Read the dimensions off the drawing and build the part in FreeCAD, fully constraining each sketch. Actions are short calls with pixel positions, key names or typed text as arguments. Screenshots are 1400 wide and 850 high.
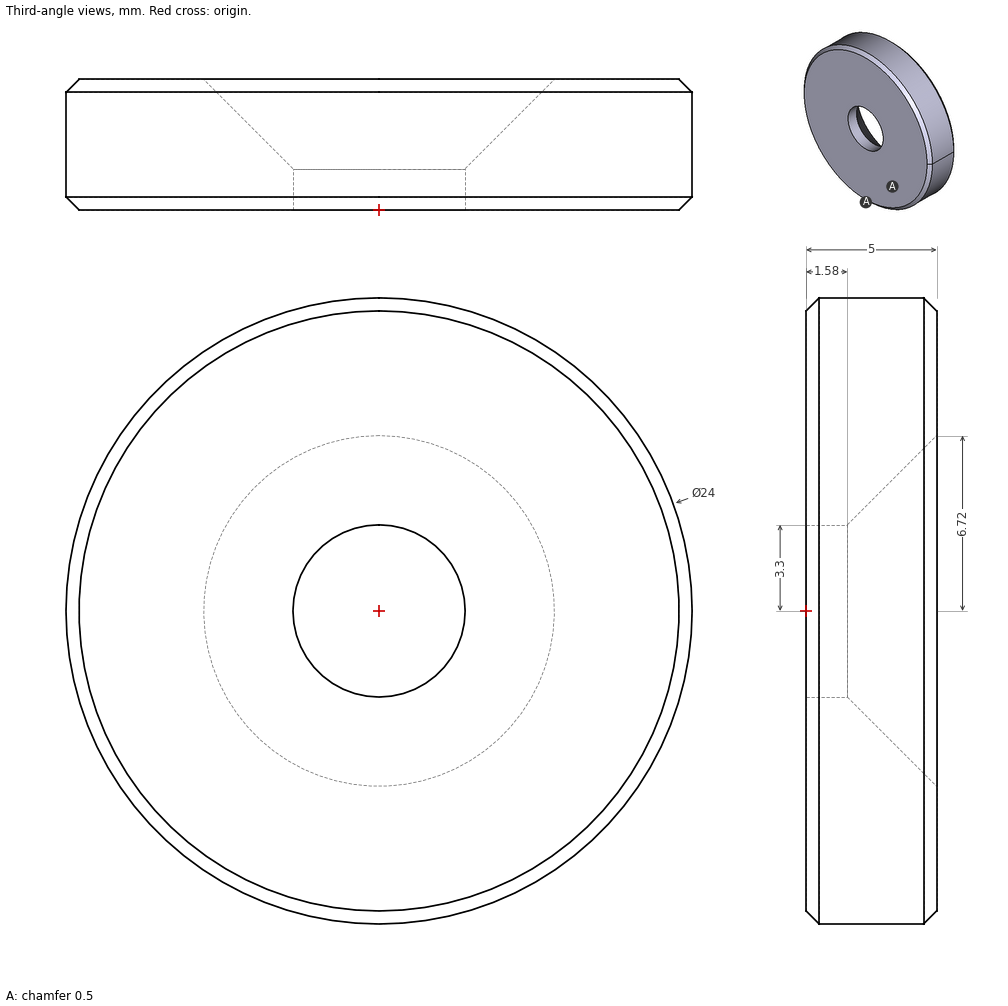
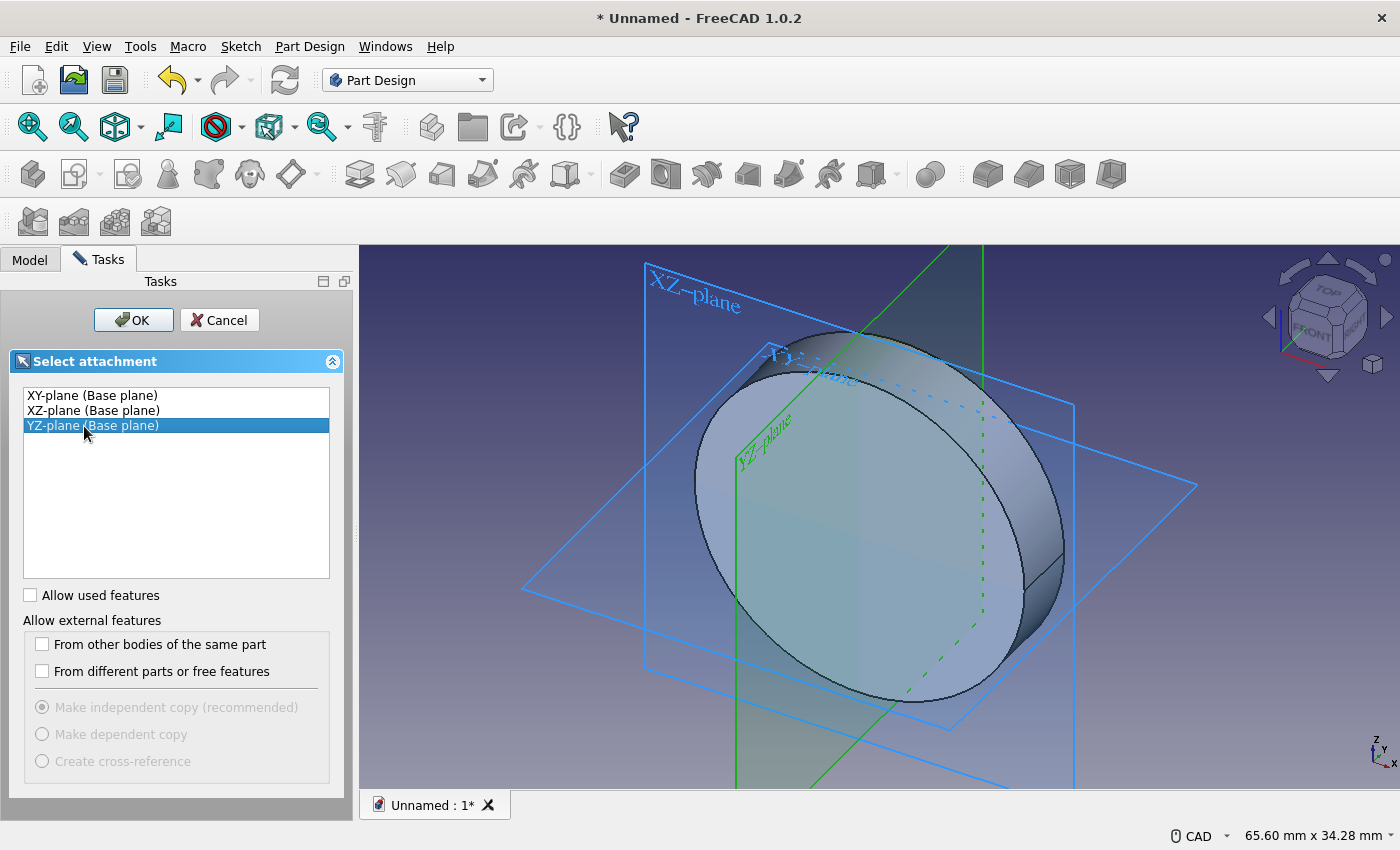
click(134, 320)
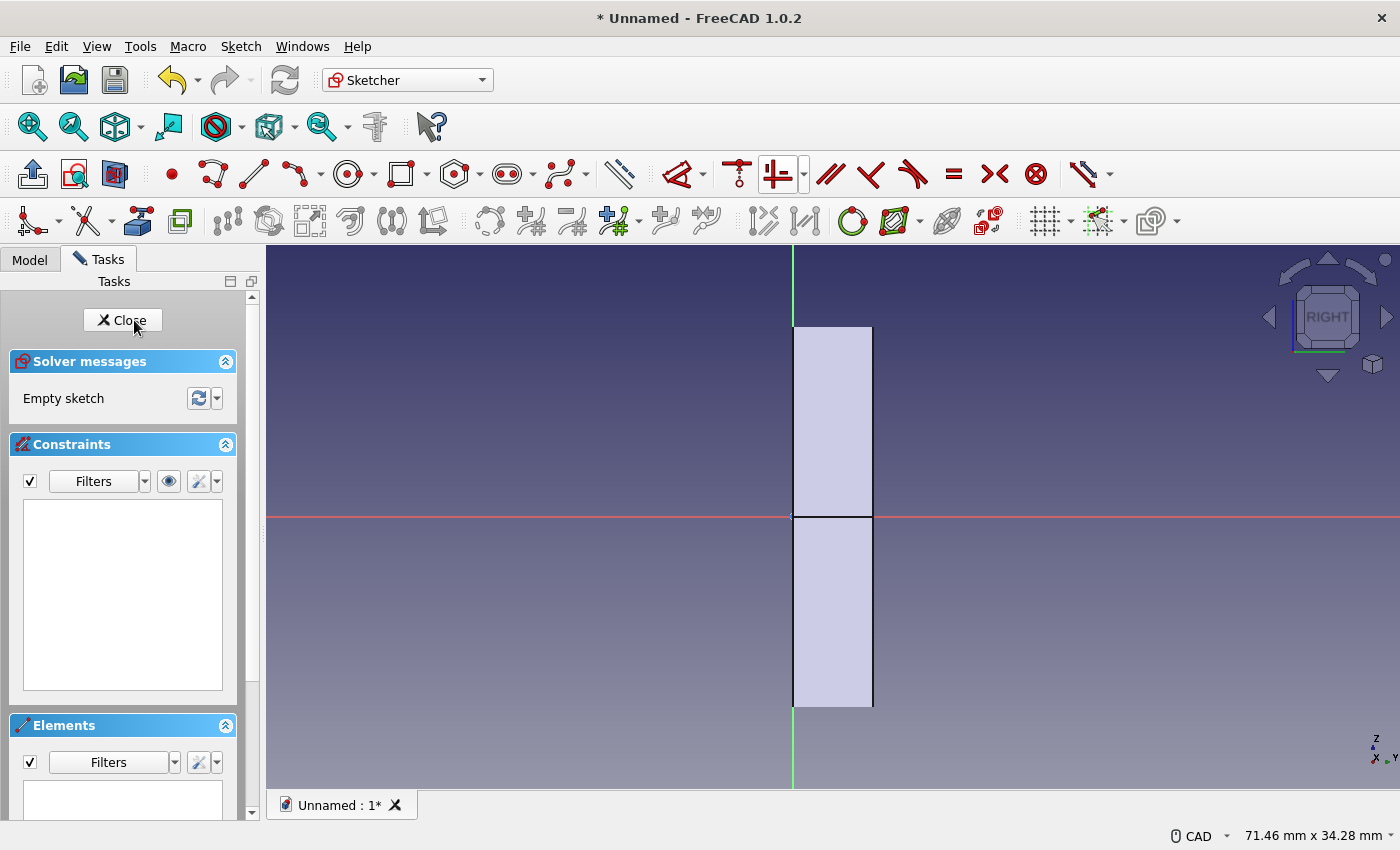
click(115, 174)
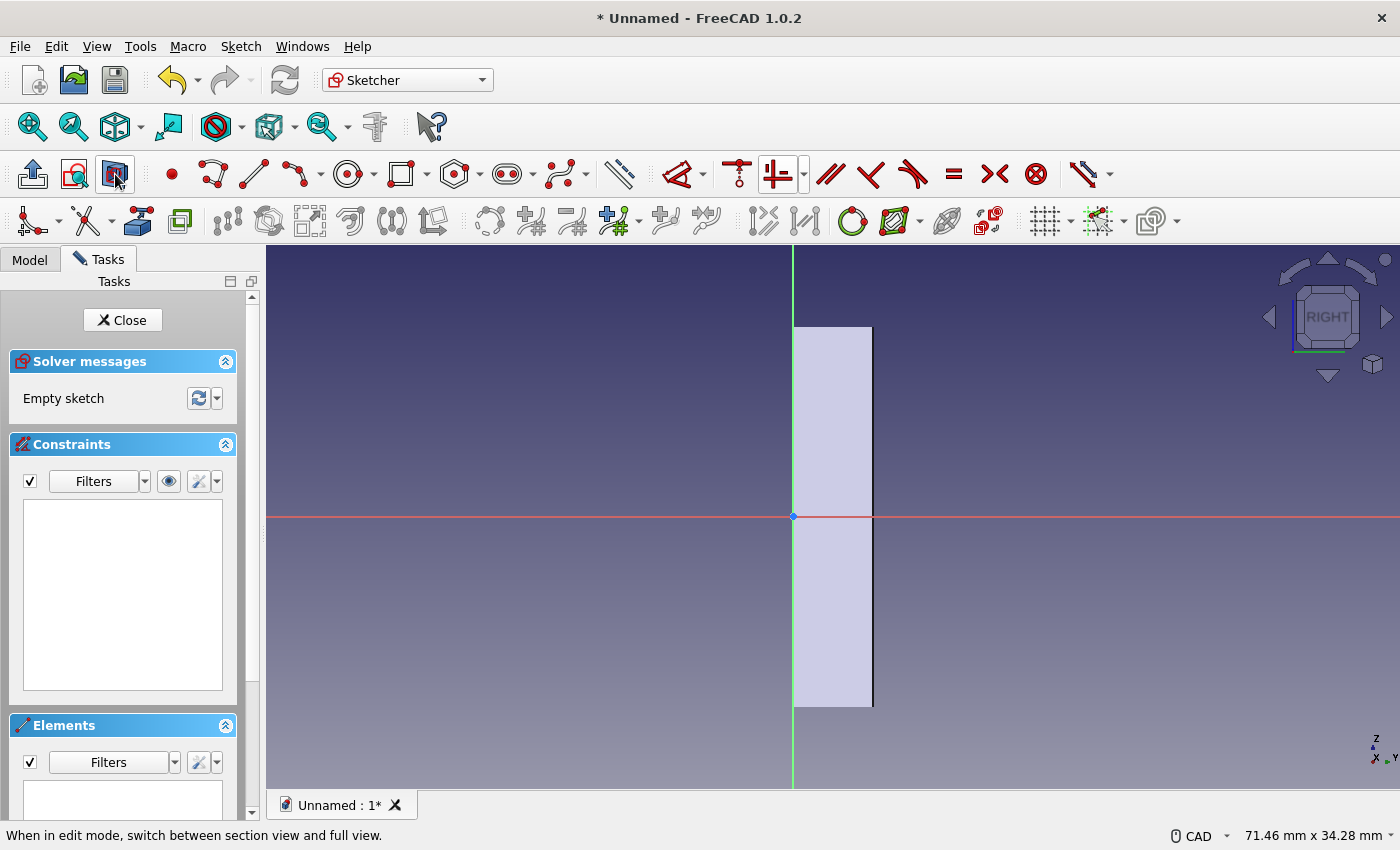
scroll(863, 441, up, 6)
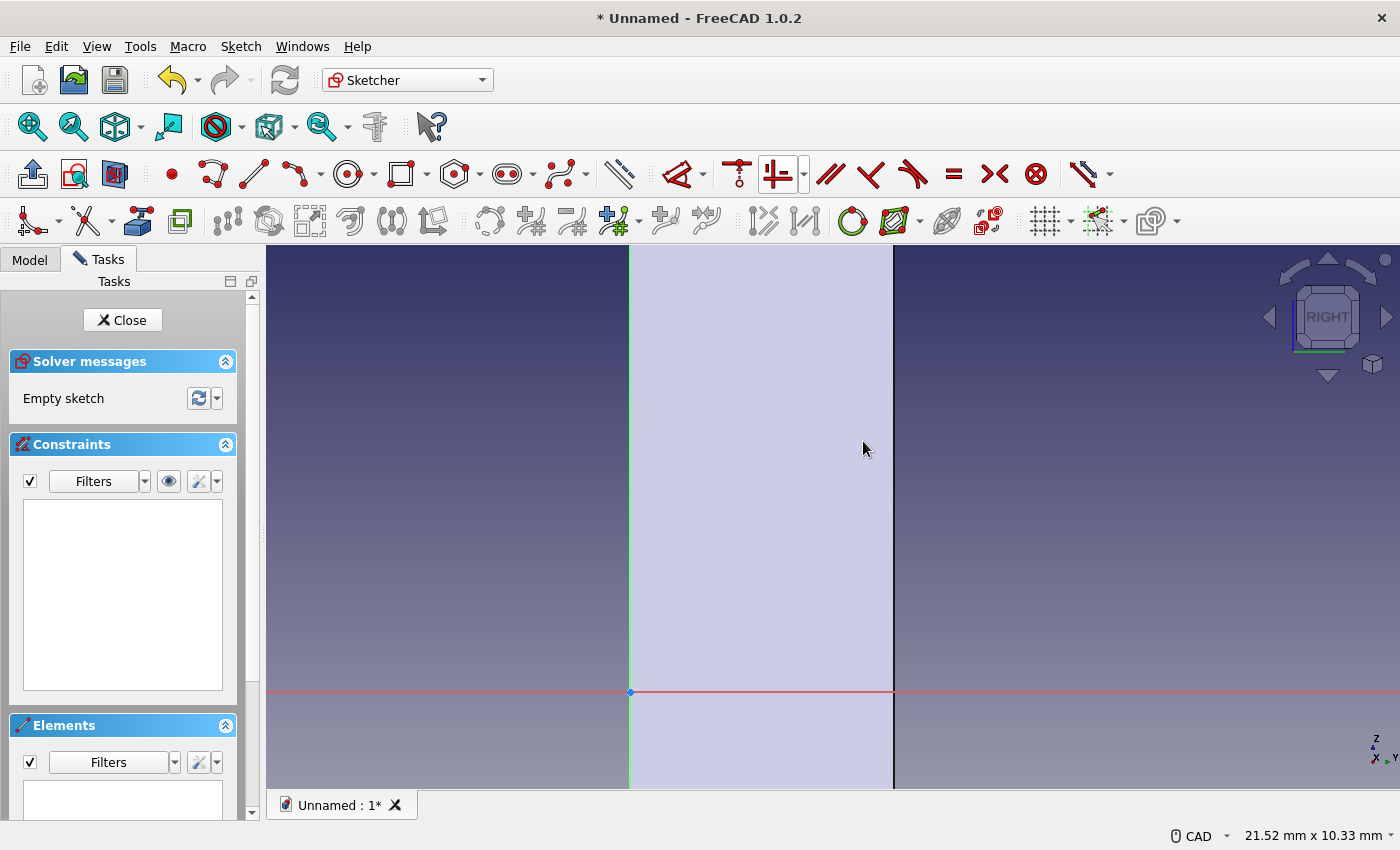
click(213, 174)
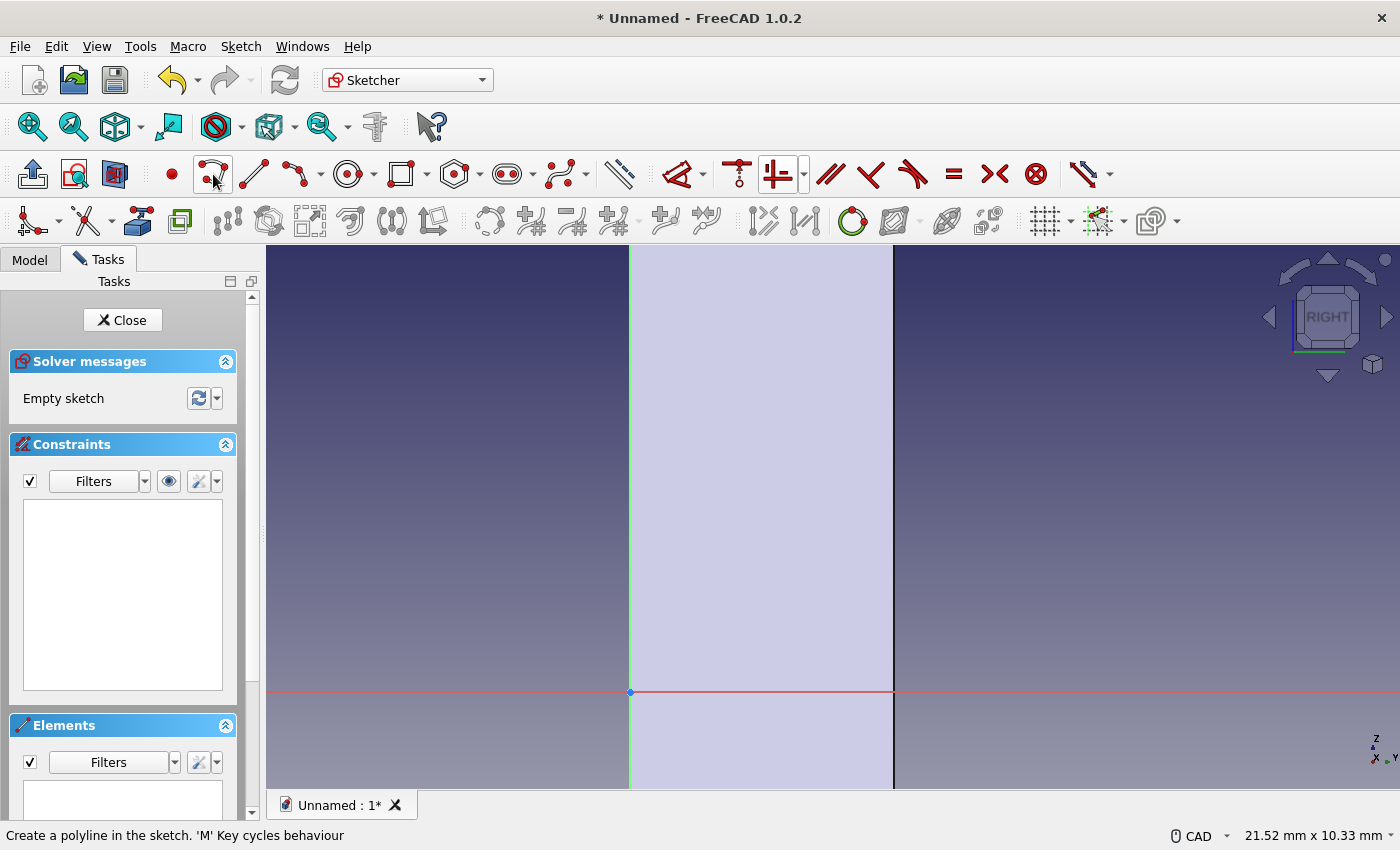
click(630, 692)
click(894, 683)
click(894, 338)
click(714, 519)
click(639, 519)
click(630, 692)
key(Escape)
key(Escape)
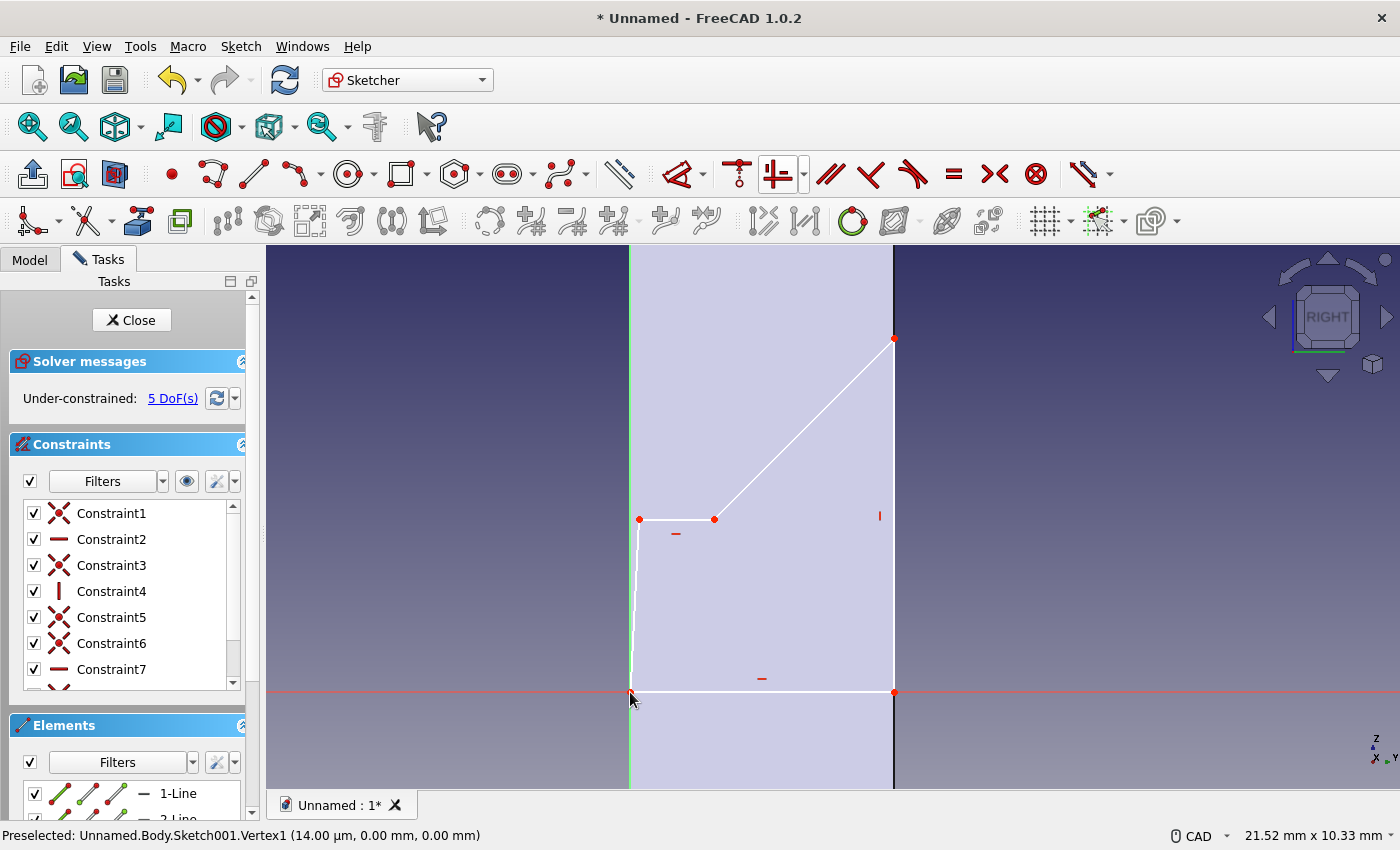
click(633, 641)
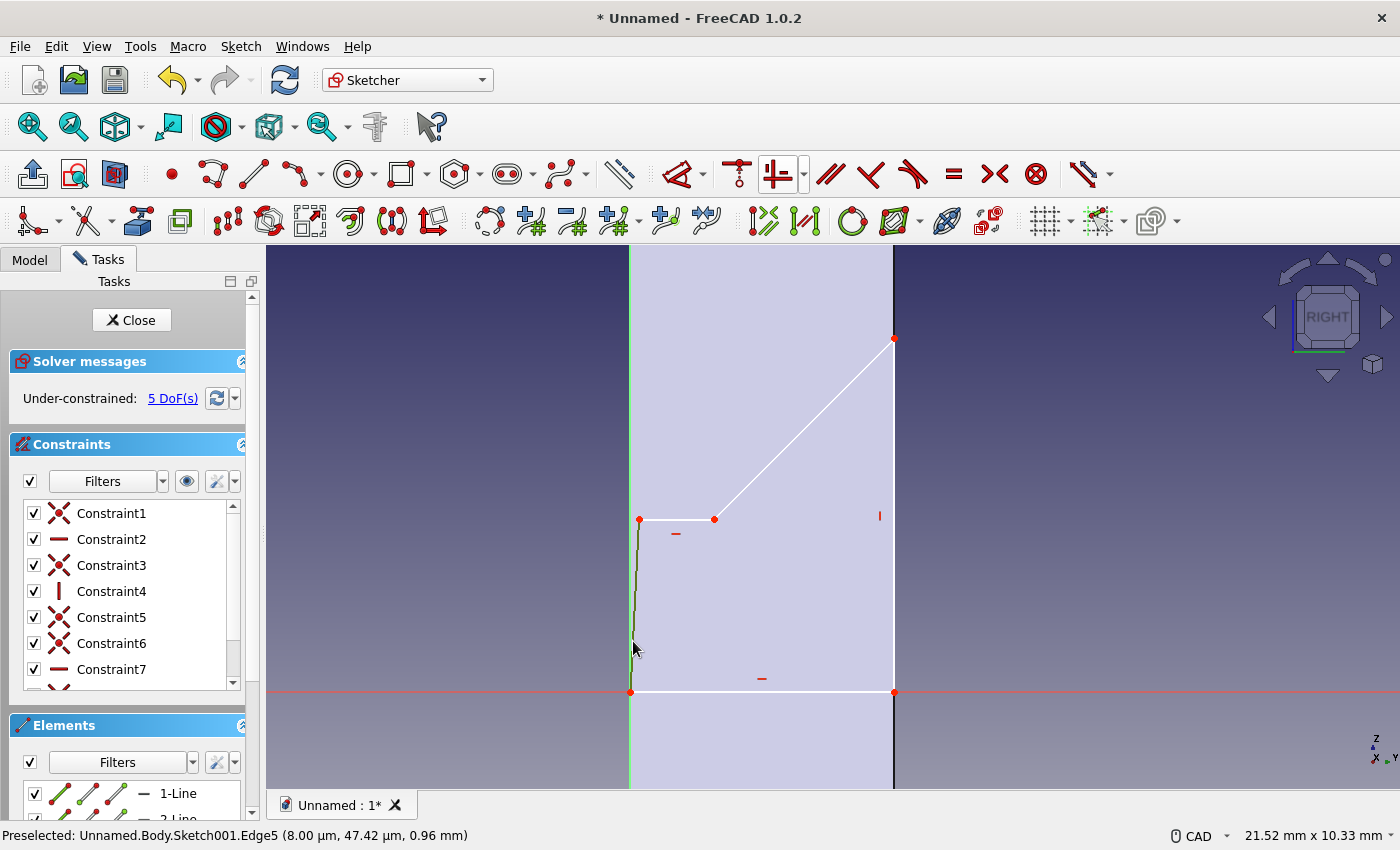
key(v)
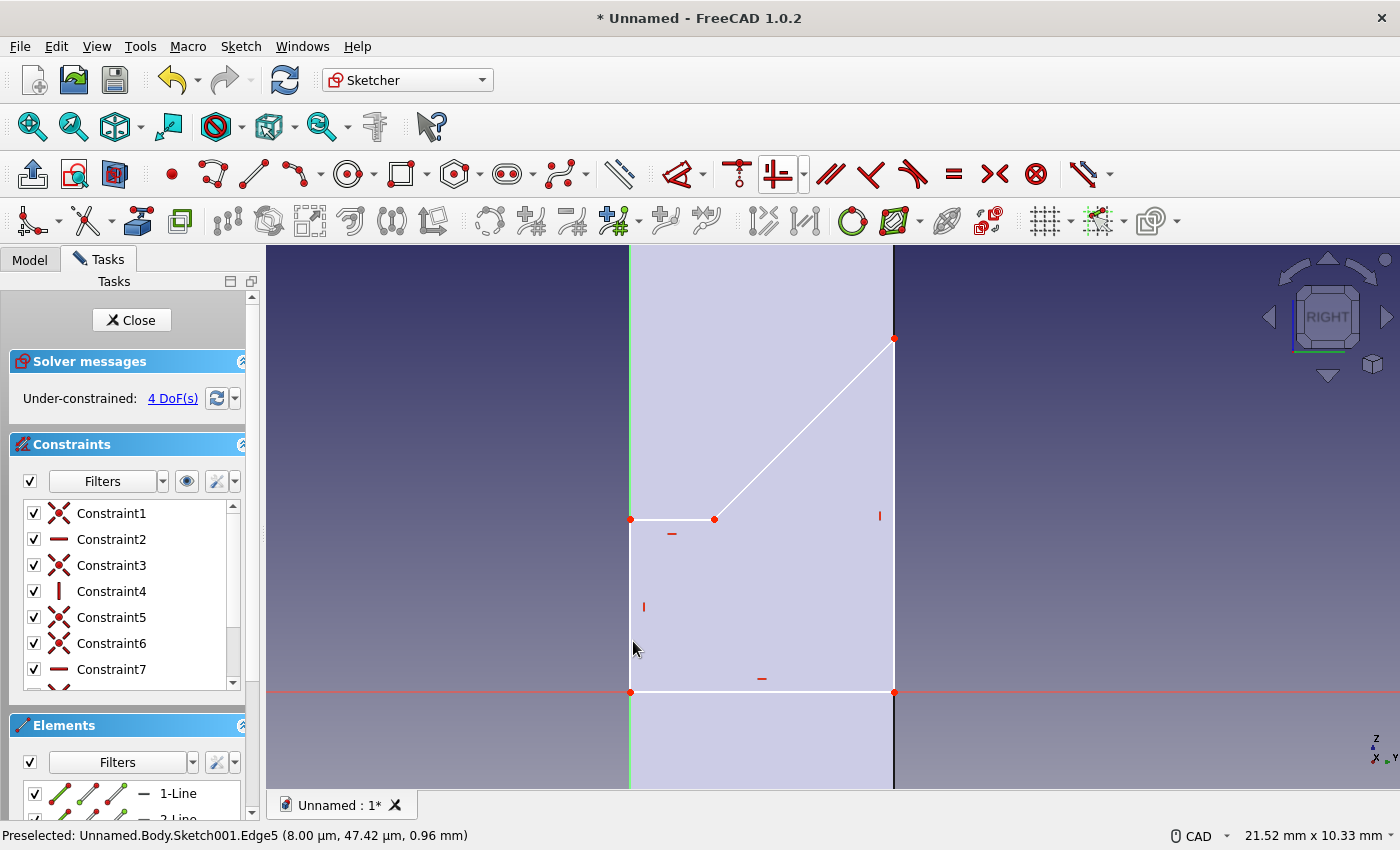
click(710, 692)